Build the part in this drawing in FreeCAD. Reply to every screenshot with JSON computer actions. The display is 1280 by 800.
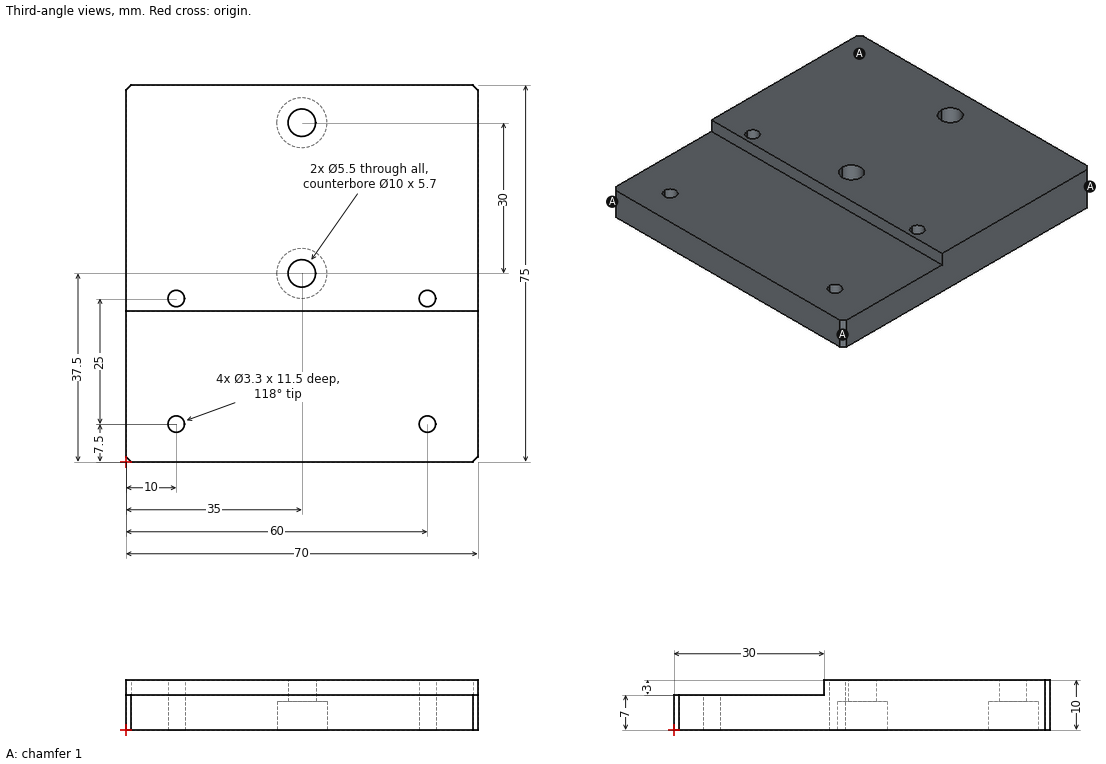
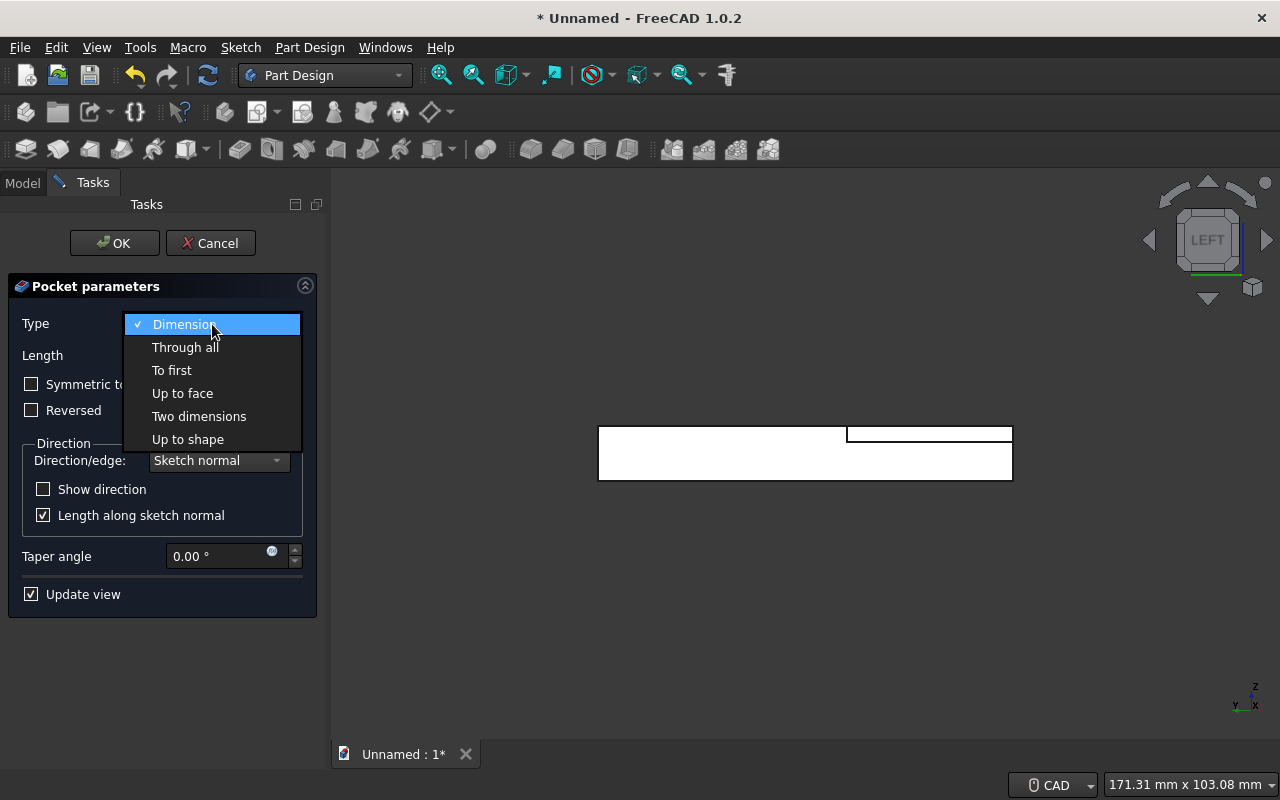
{"action": "left_click", "coordinate": [212, 348]}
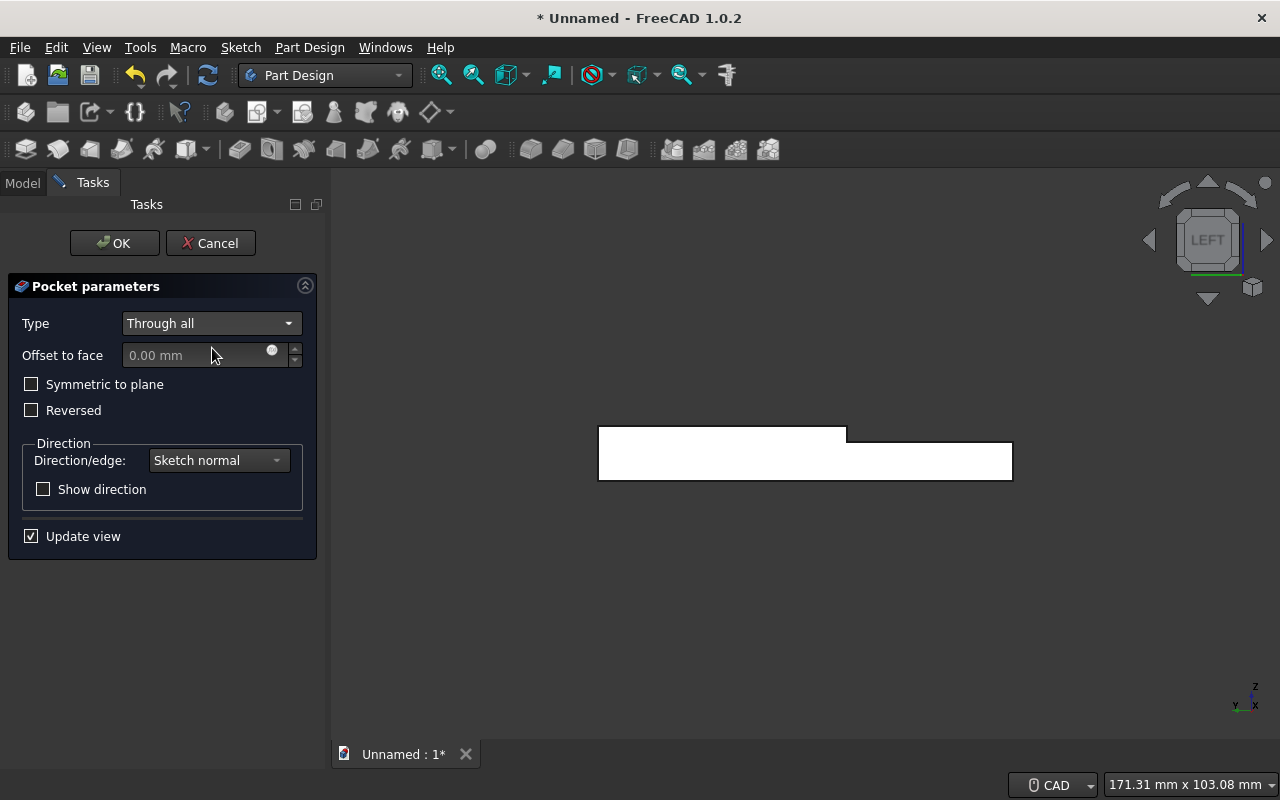
{"action": "left_click", "coordinate": [115, 243]}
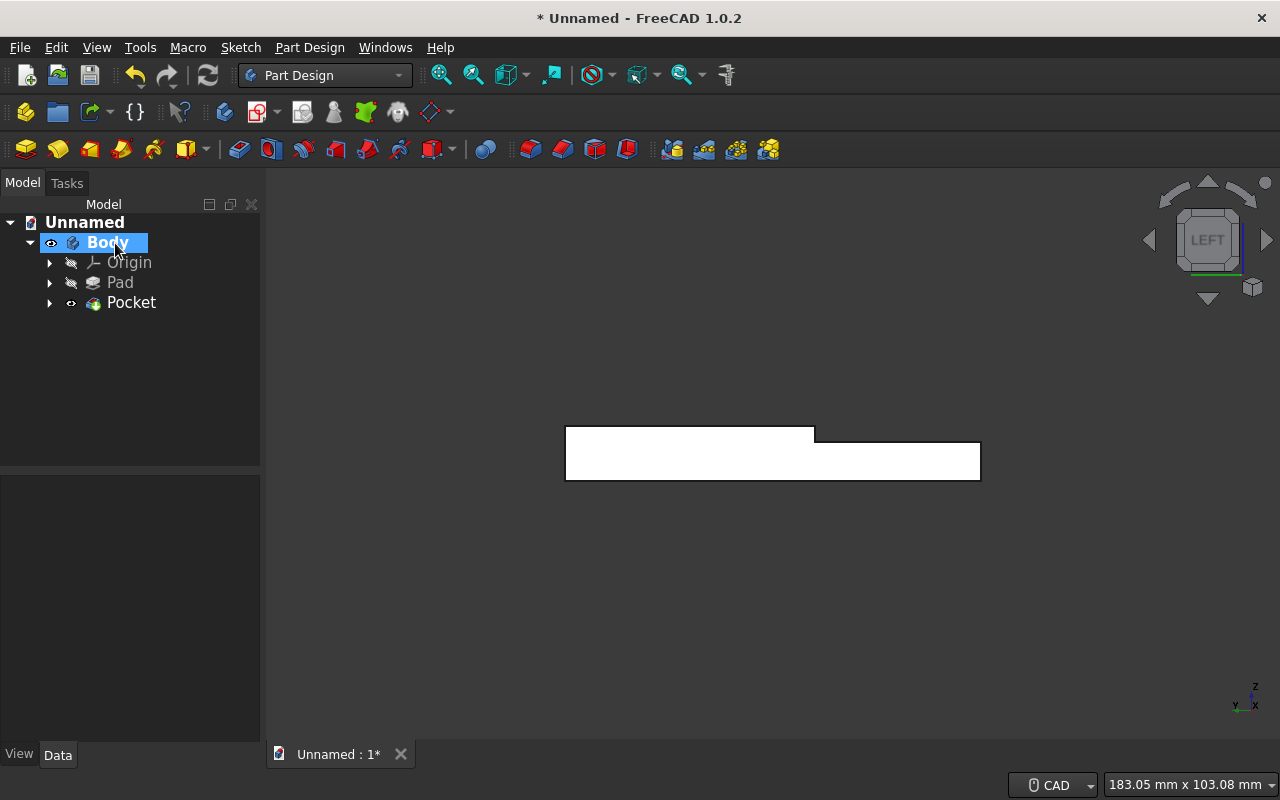
{"action": "key", "text": "v f"}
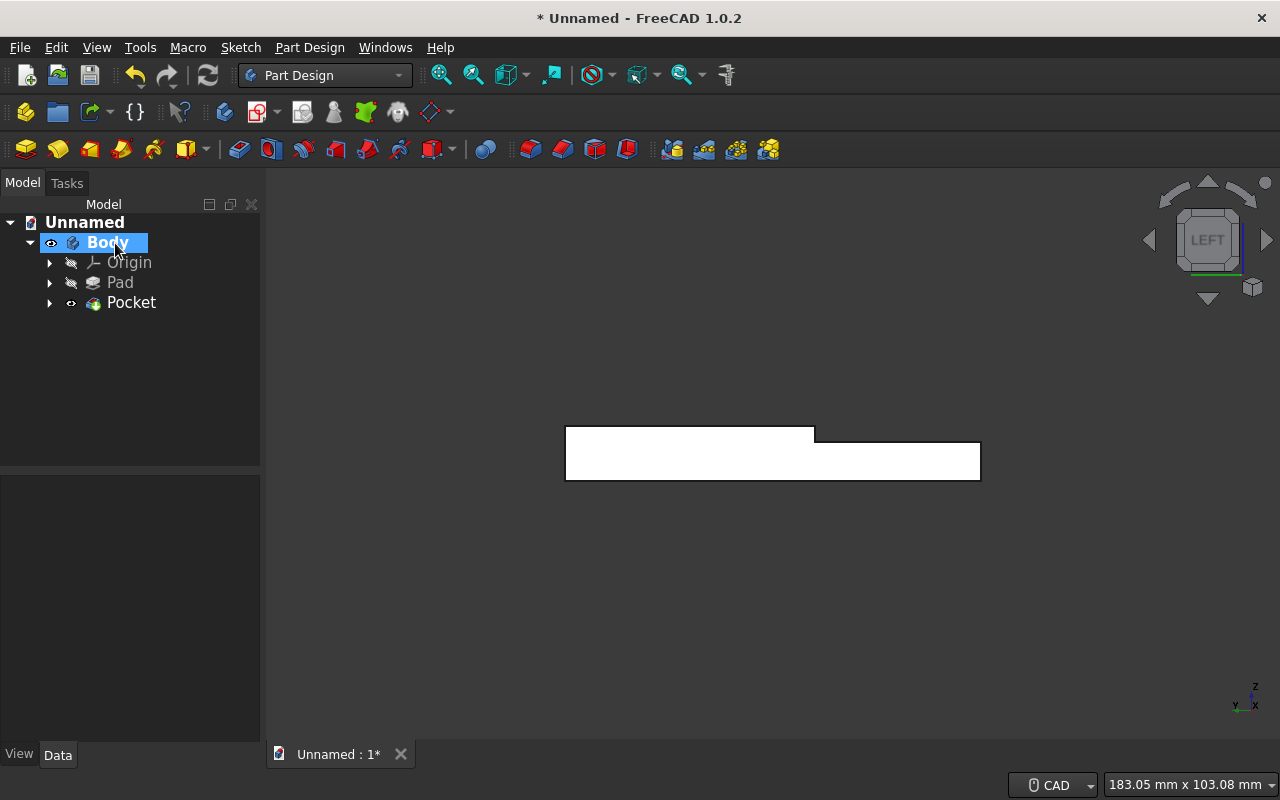
{"action": "key", "text": "5"}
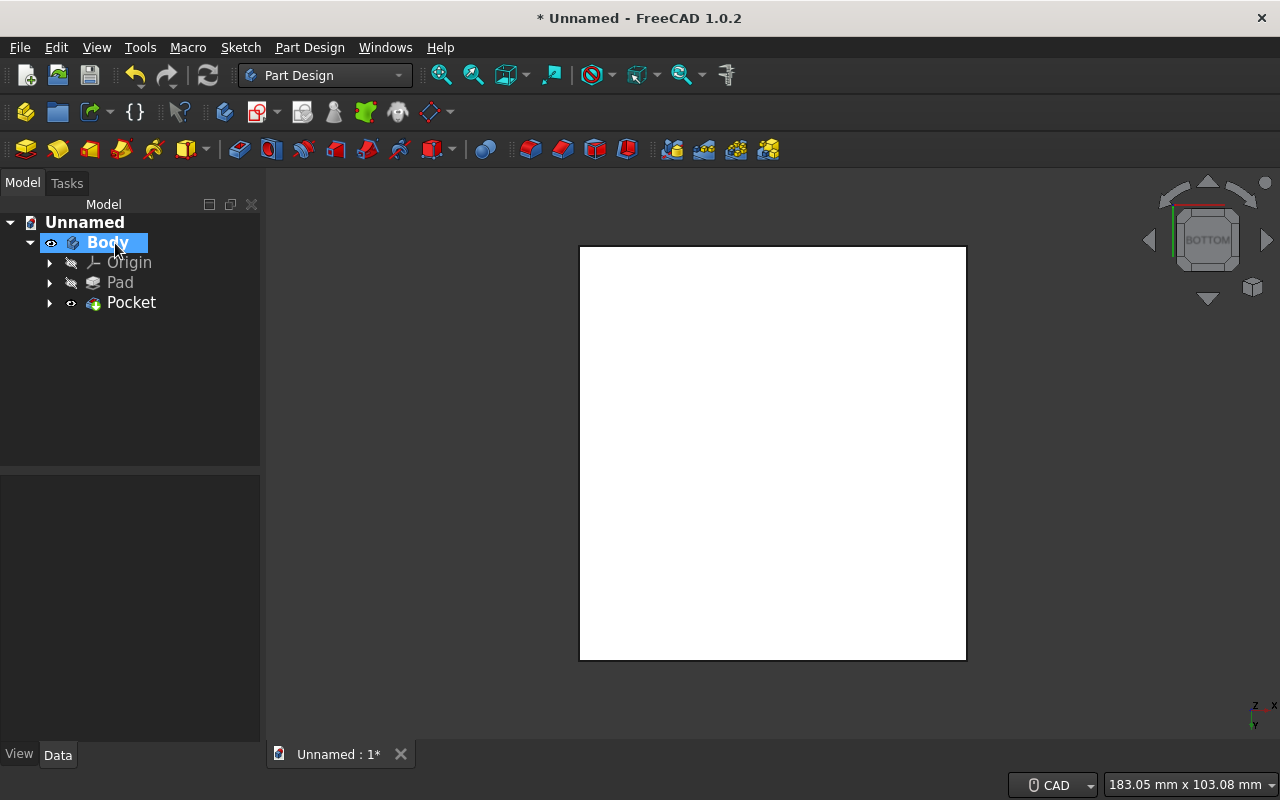
{"action": "left_click", "coordinate": [773, 452]}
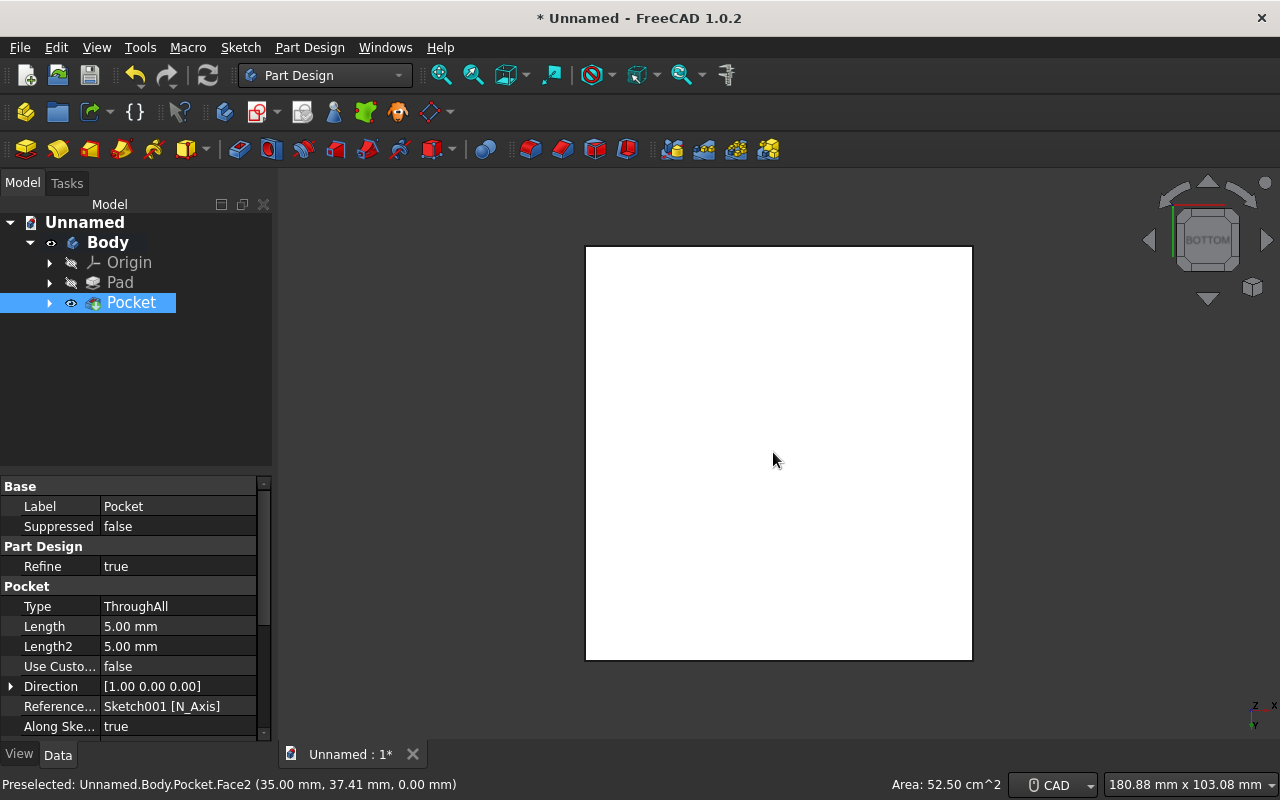
{"action": "left_click", "coordinate": [258, 112]}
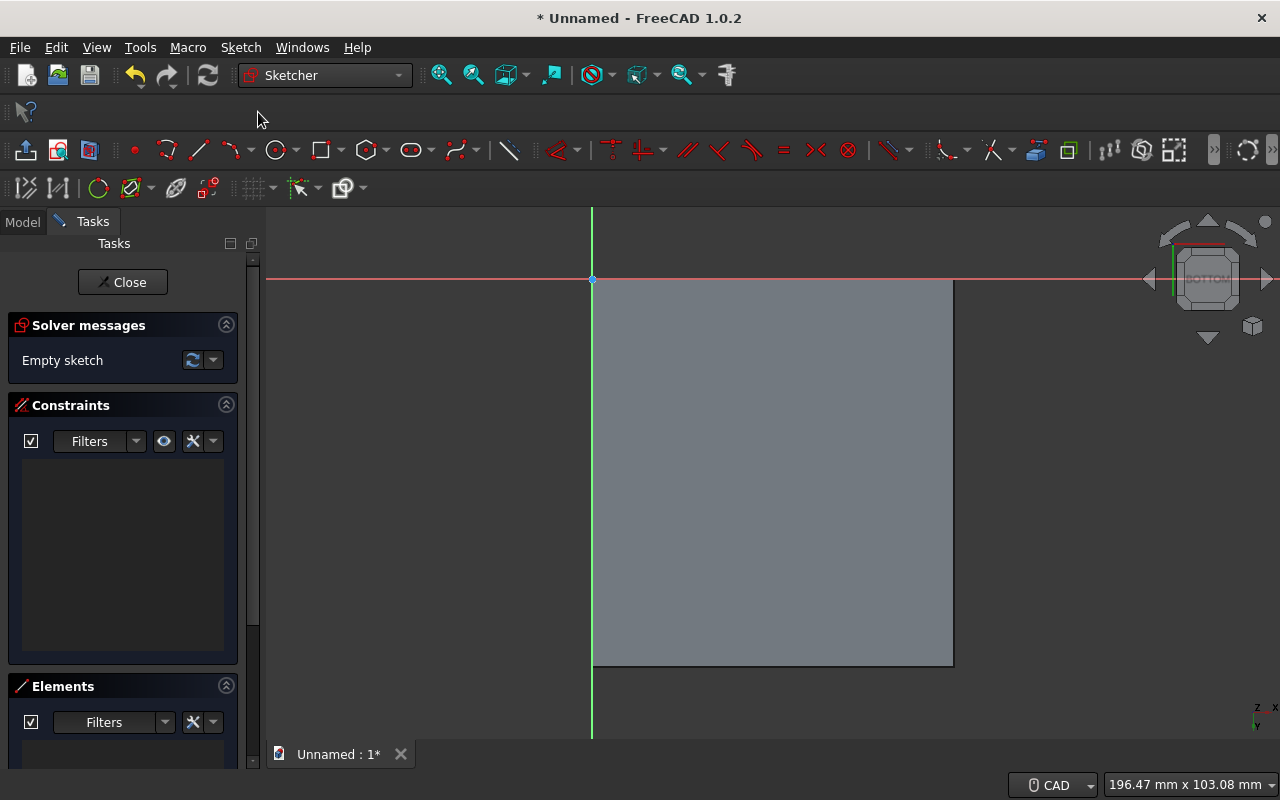
{"action": "scroll", "coordinate": [809, 239], "scroll_direction": "up", "scroll_amount": 3}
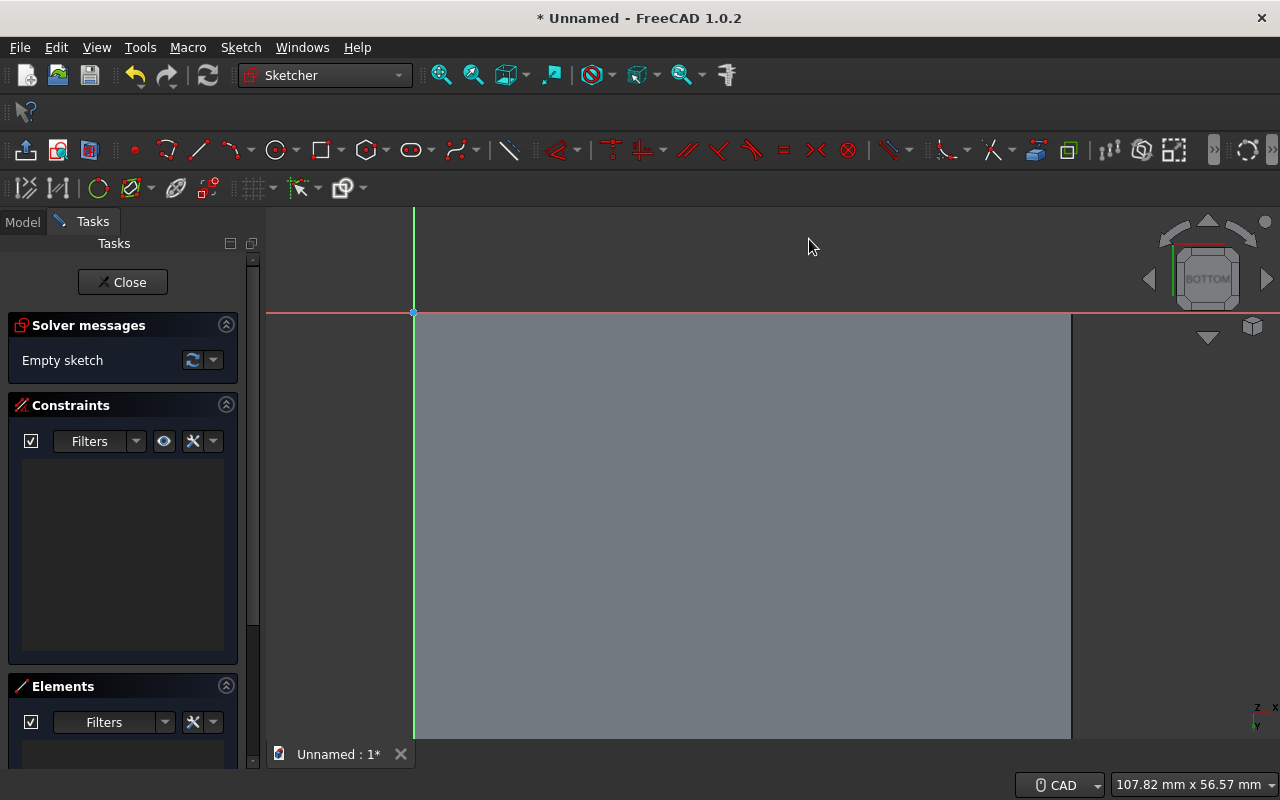
{"action": "left_click", "coordinate": [276, 150]}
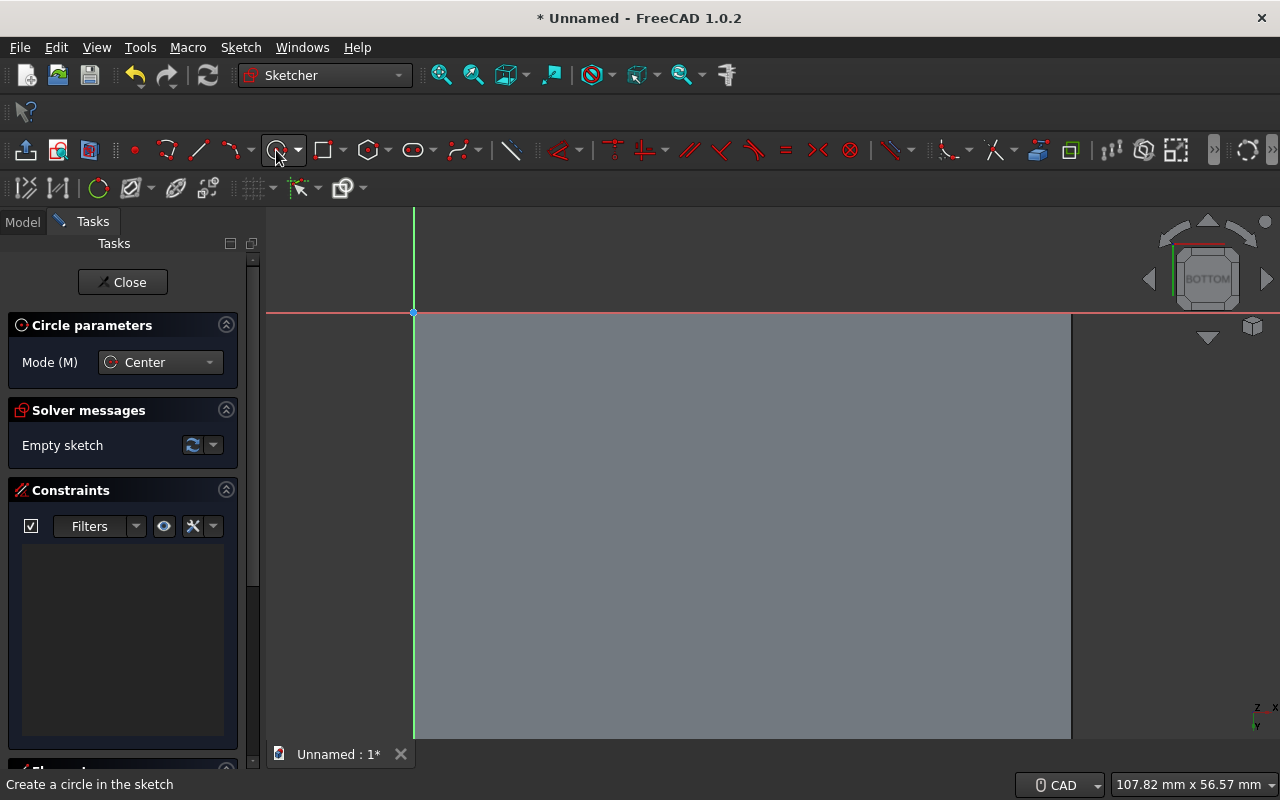
{"action": "scroll", "coordinate": [508, 383], "scroll_direction": "up", "scroll_amount": 2}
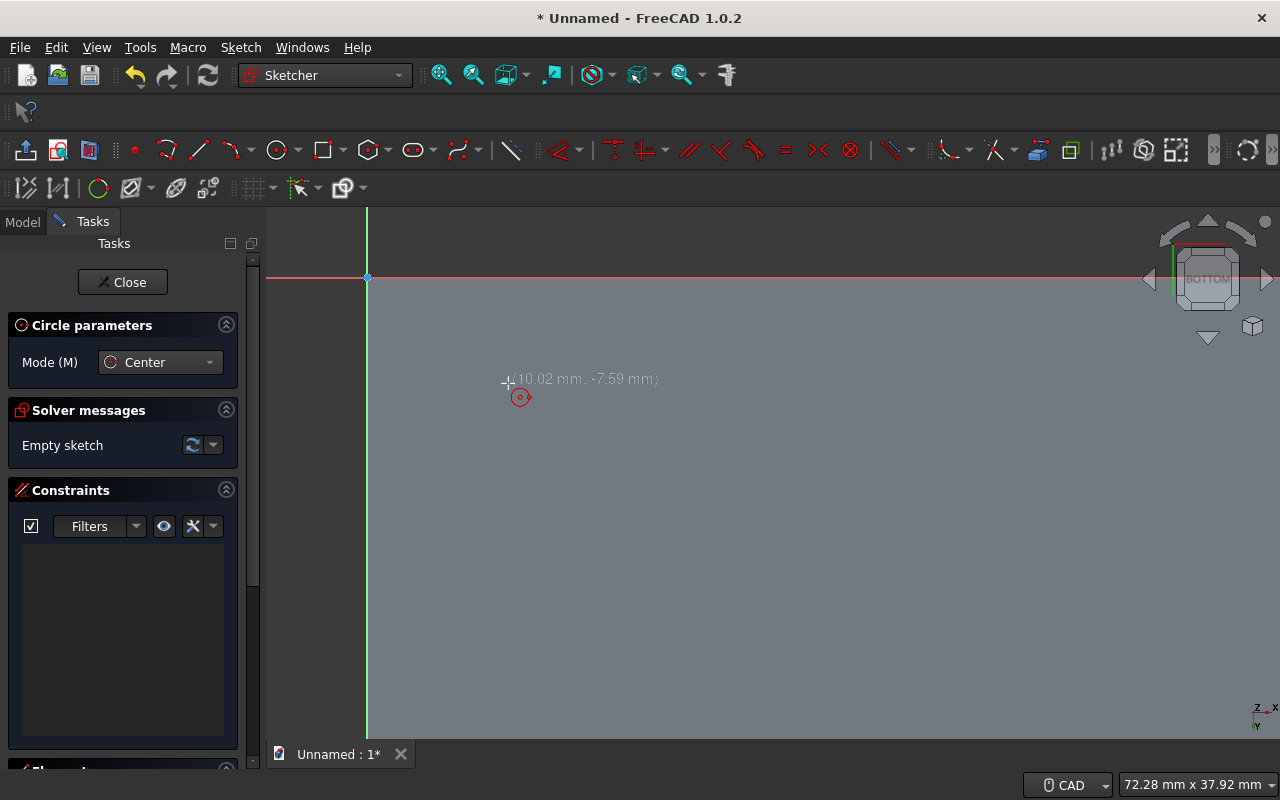
{"action": "left_click", "coordinate": [508, 383]}
{"action": "mouse_move", "coordinate": [524, 367]}